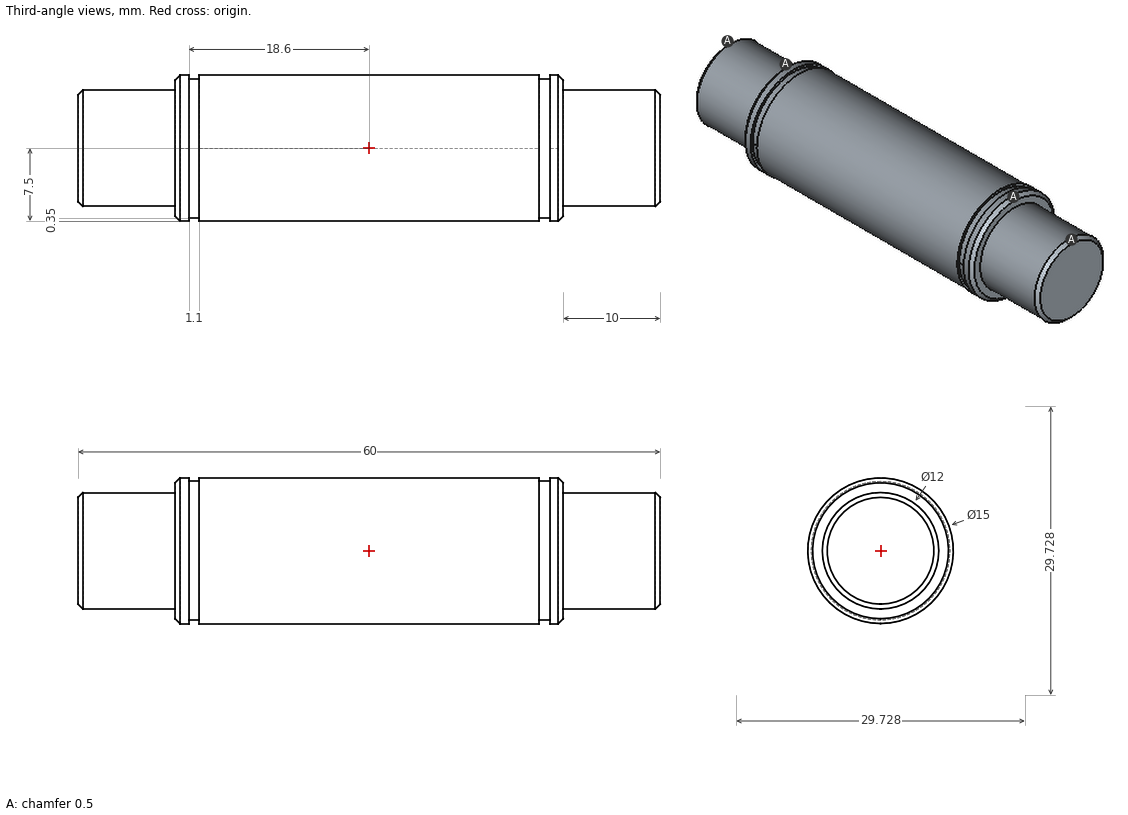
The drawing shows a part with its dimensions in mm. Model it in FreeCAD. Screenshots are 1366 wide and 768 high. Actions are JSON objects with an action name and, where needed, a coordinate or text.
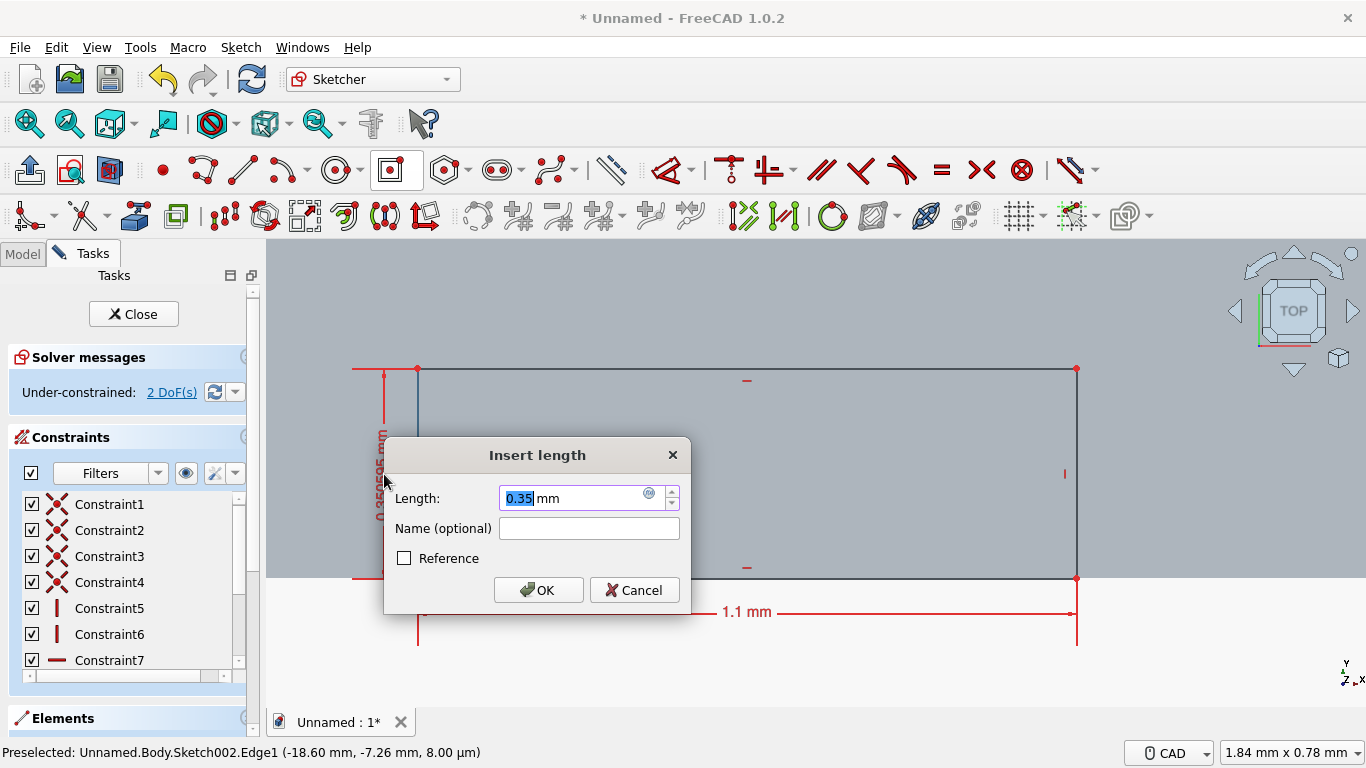
{"action": "type", "text": "0.35"}
{"action": "key", "text": "Return"}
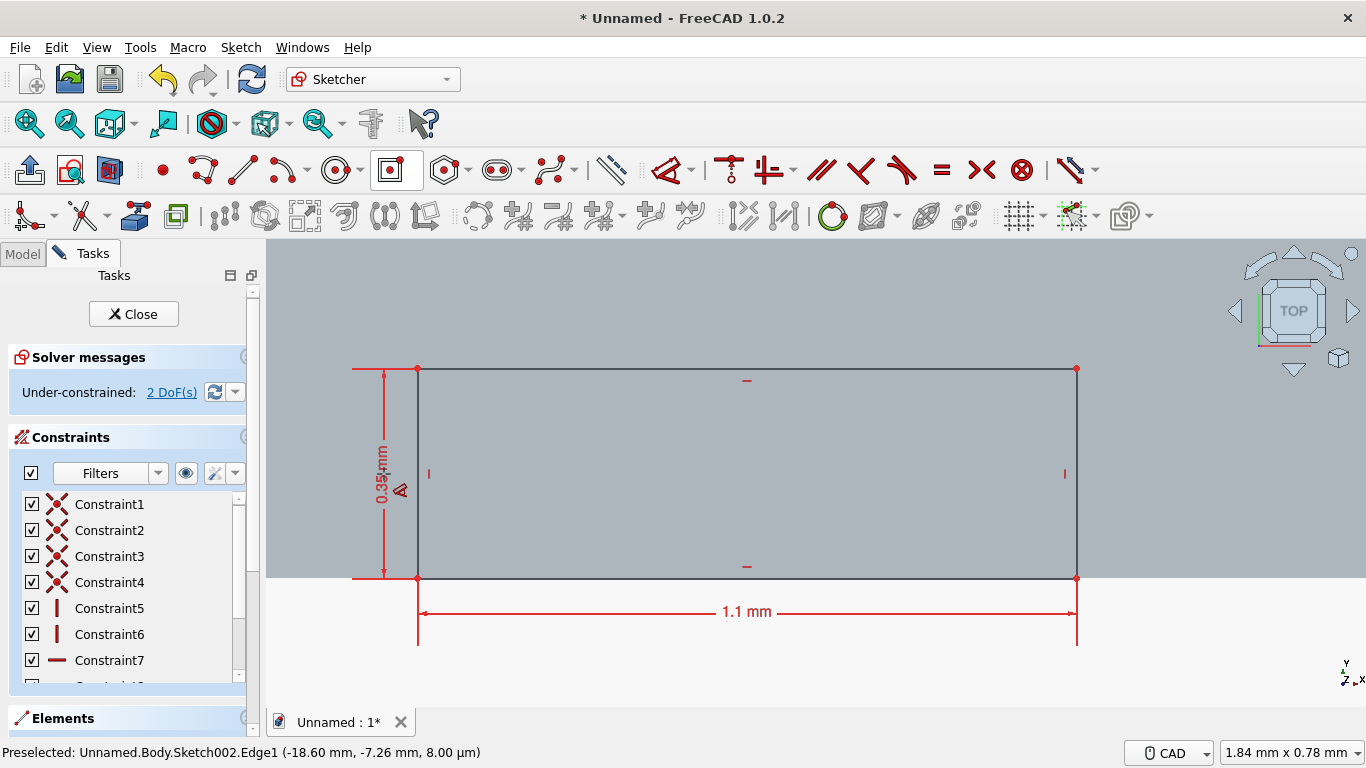
{"action": "left_click", "coordinate": [418, 579]}
{"action": "left_click", "coordinate": [384, 423]}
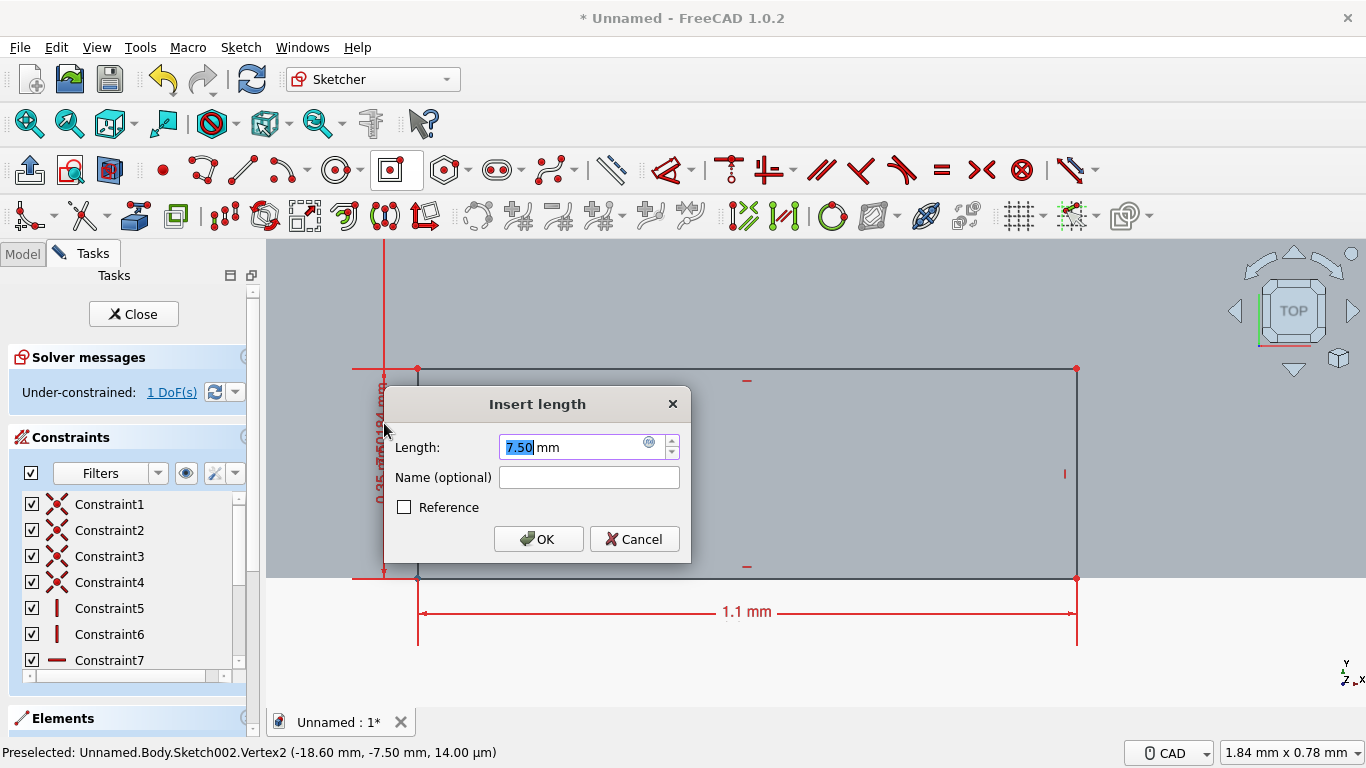
{"action": "type", "text": "7.5"}
{"action": "key", "text": "Return"}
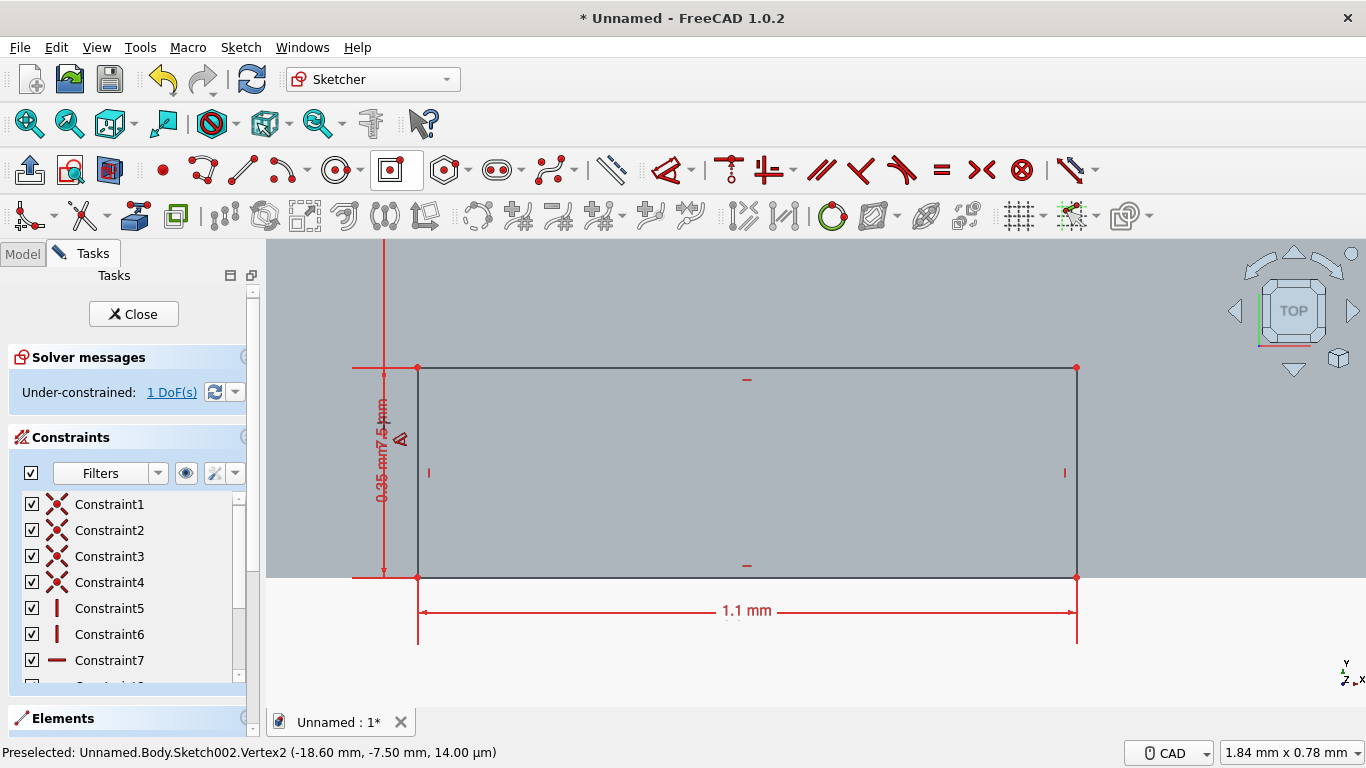
{"action": "left_click", "coordinate": [418, 368]}
{"action": "left_click", "coordinate": [809, 402]}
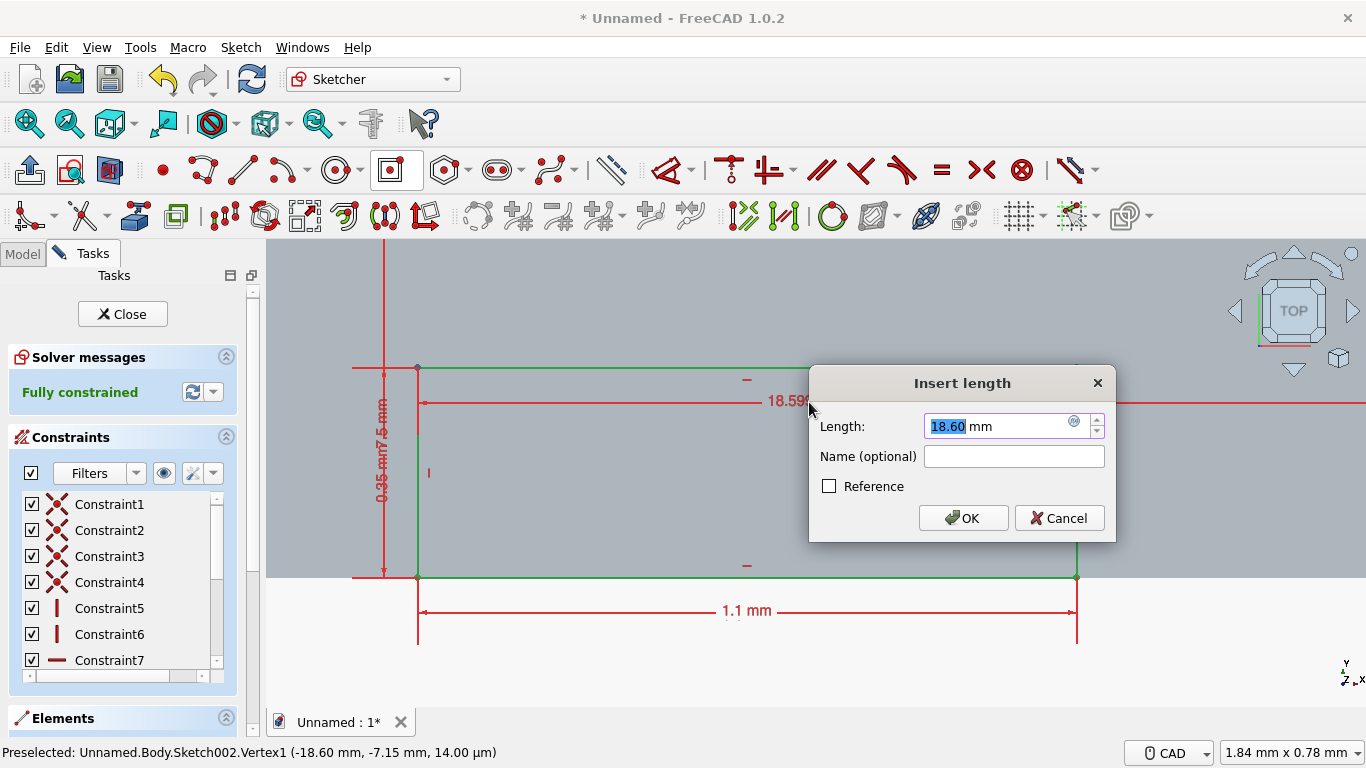
{"action": "type", "text": "18.6"}
{"action": "key", "text": "Return"}
{"action": "key", "text": "Escape"}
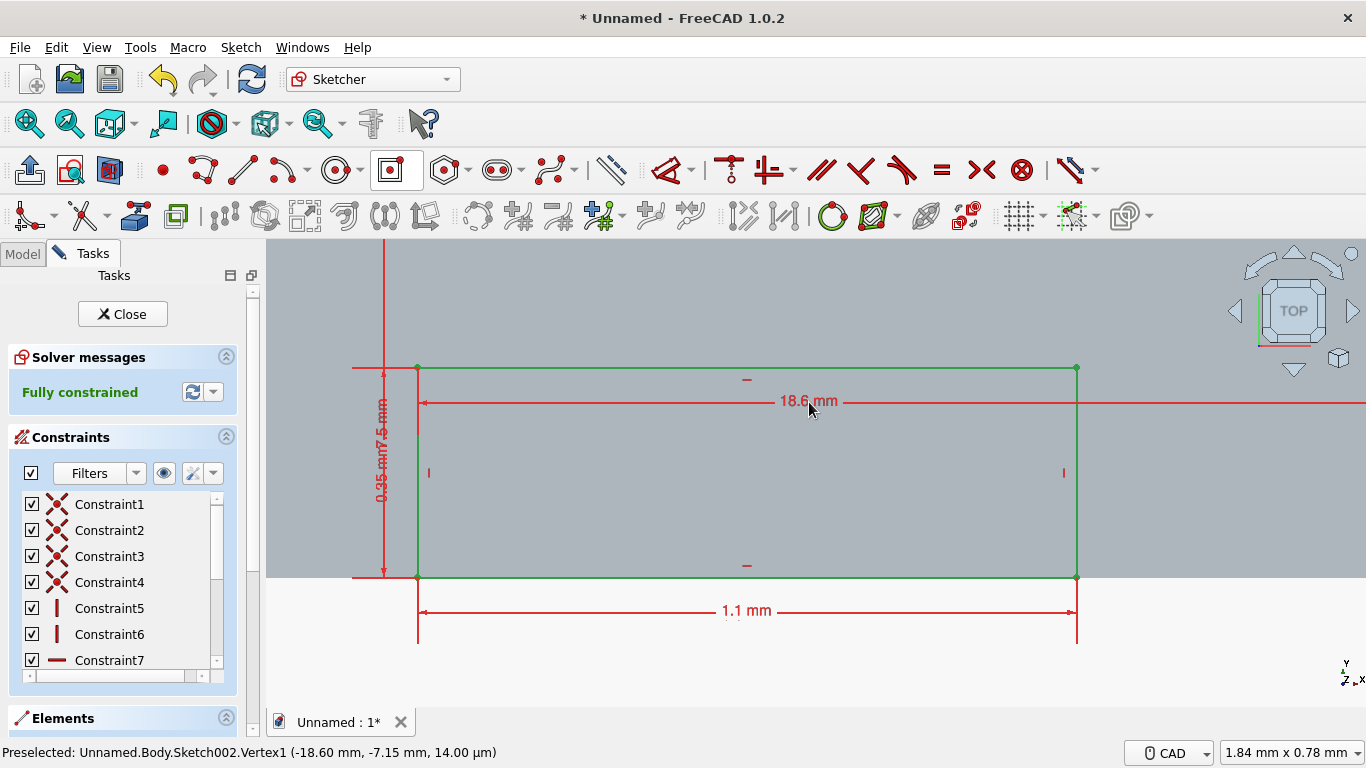
{"action": "left_click", "coordinate": [123, 314]}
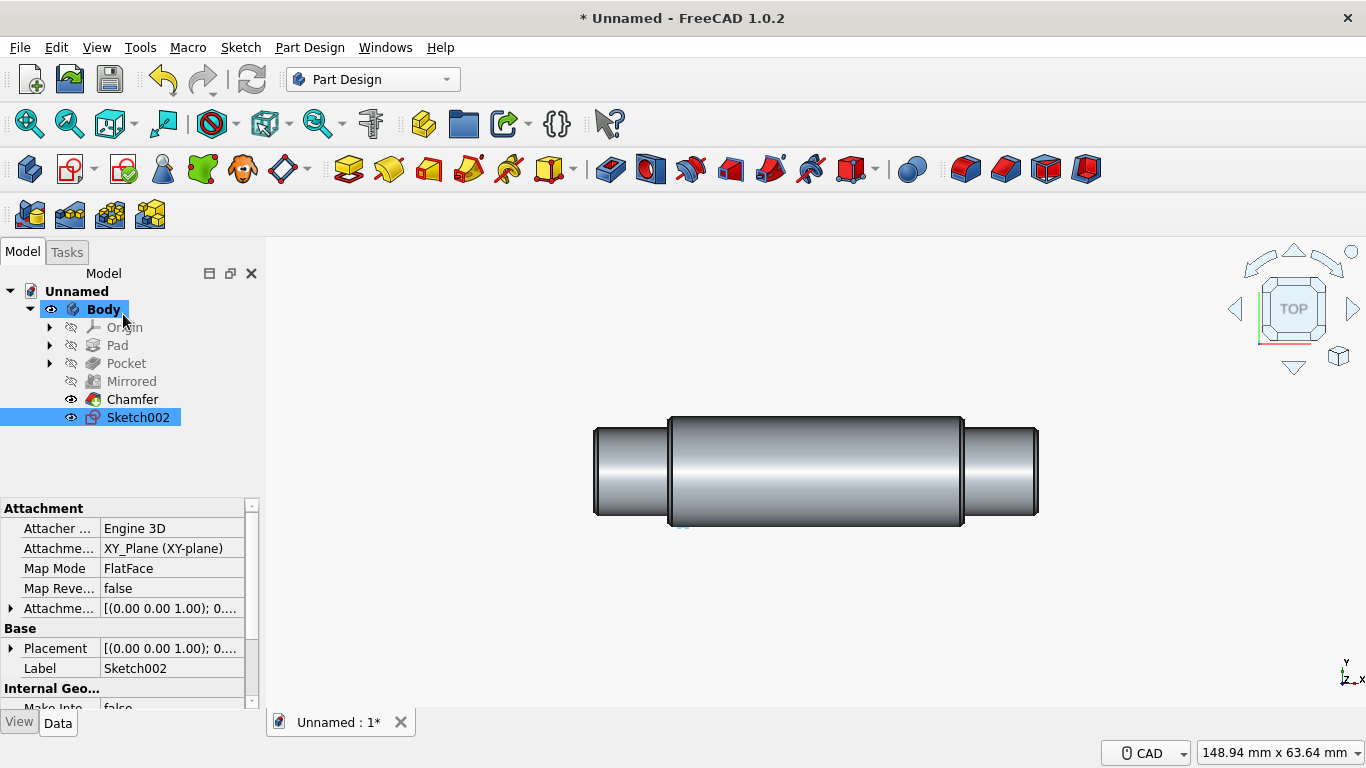
{"action": "left_click", "coordinate": [692, 170]}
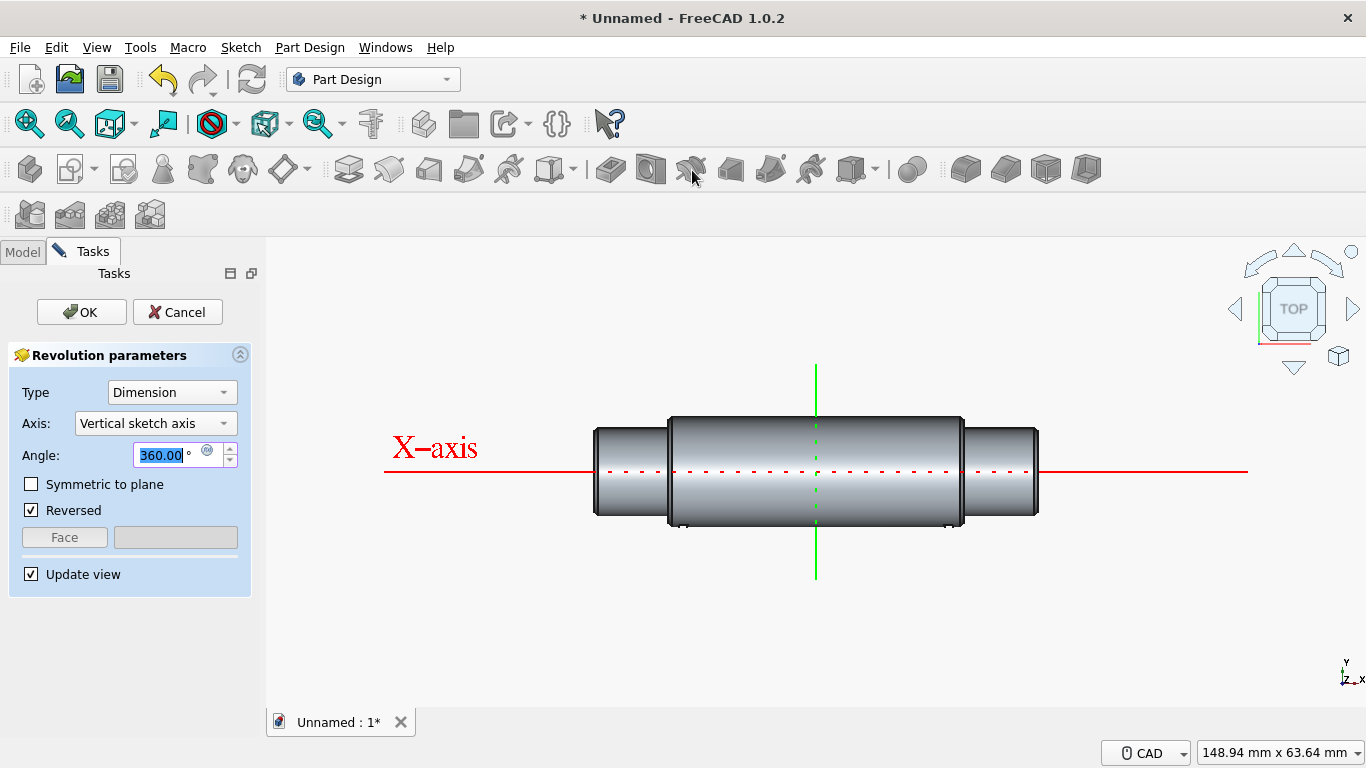
{"action": "left_click", "coordinate": [156, 424]}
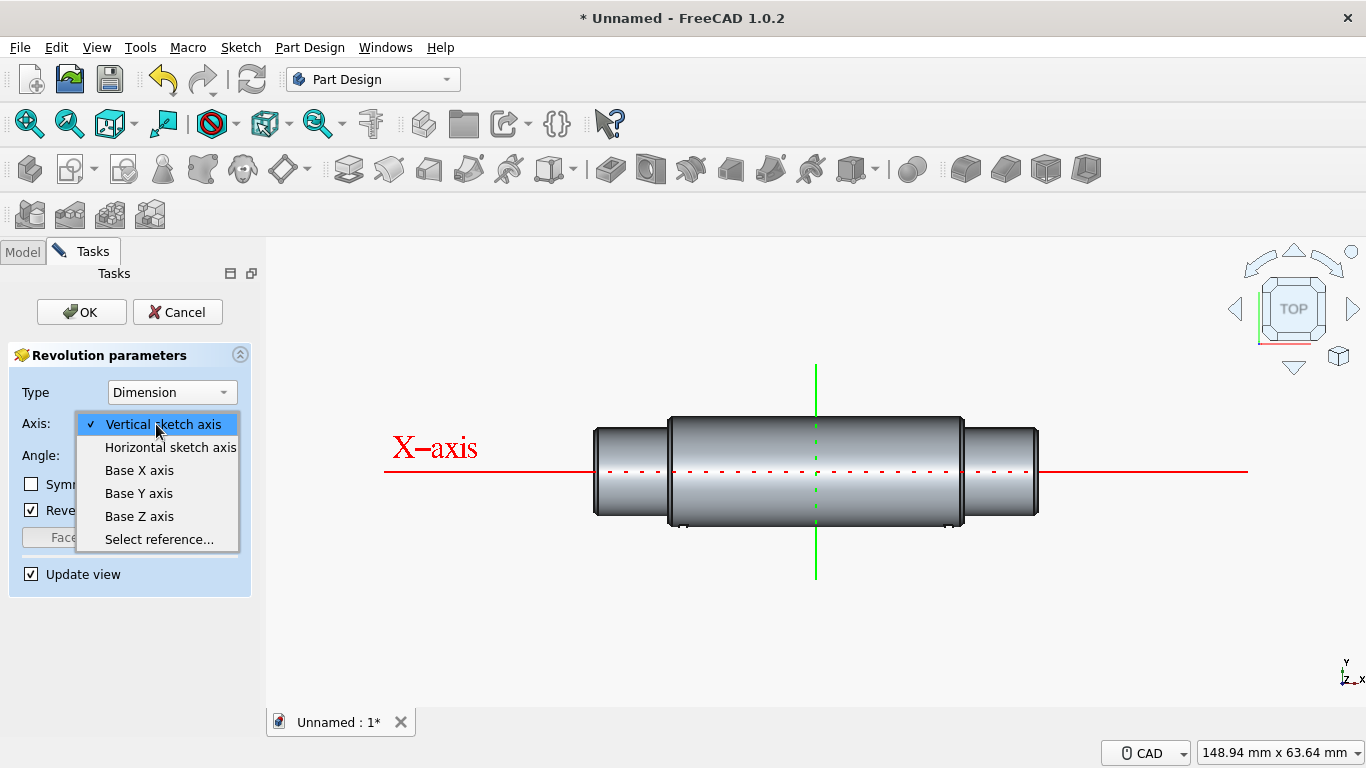
{"action": "left_click", "coordinate": [156, 448]}